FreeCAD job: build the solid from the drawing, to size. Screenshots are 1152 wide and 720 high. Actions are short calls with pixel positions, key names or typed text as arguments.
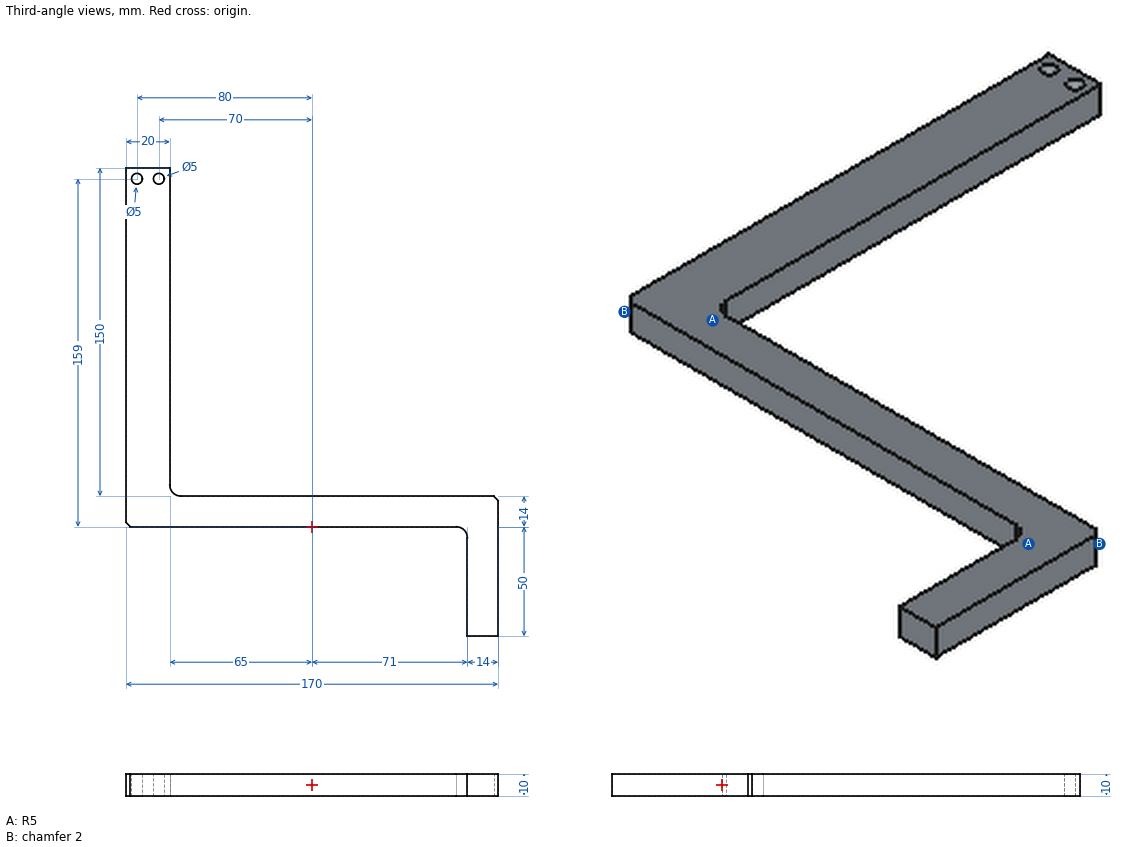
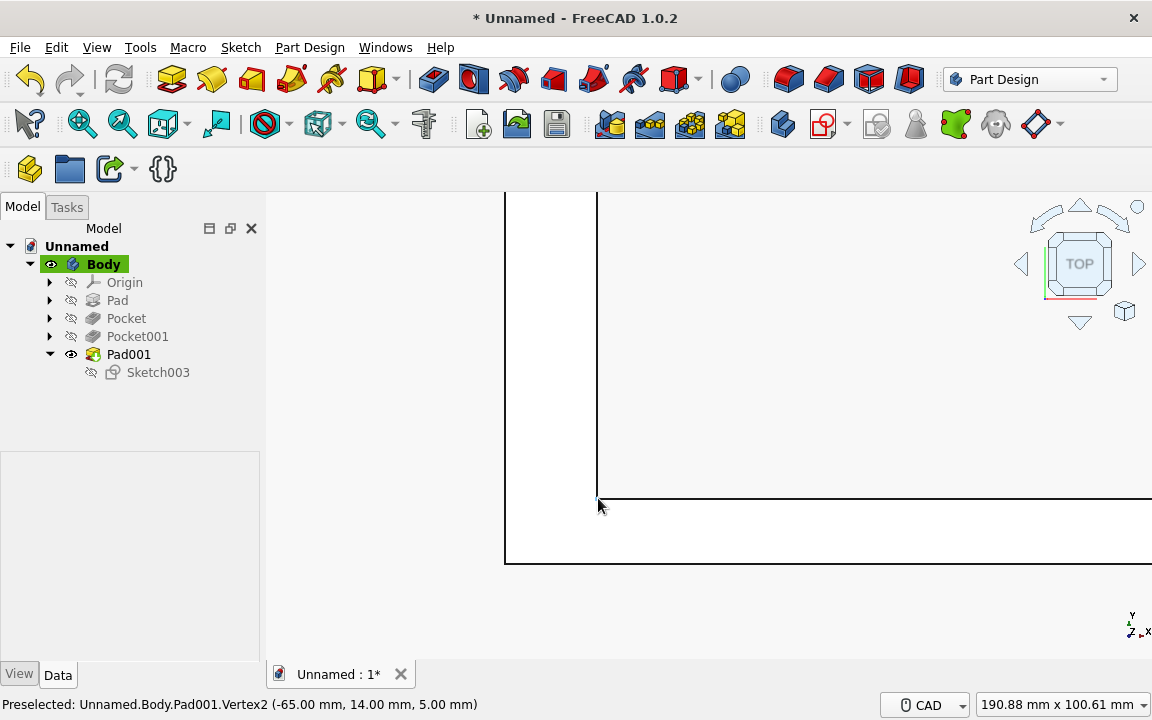
click(84, 124)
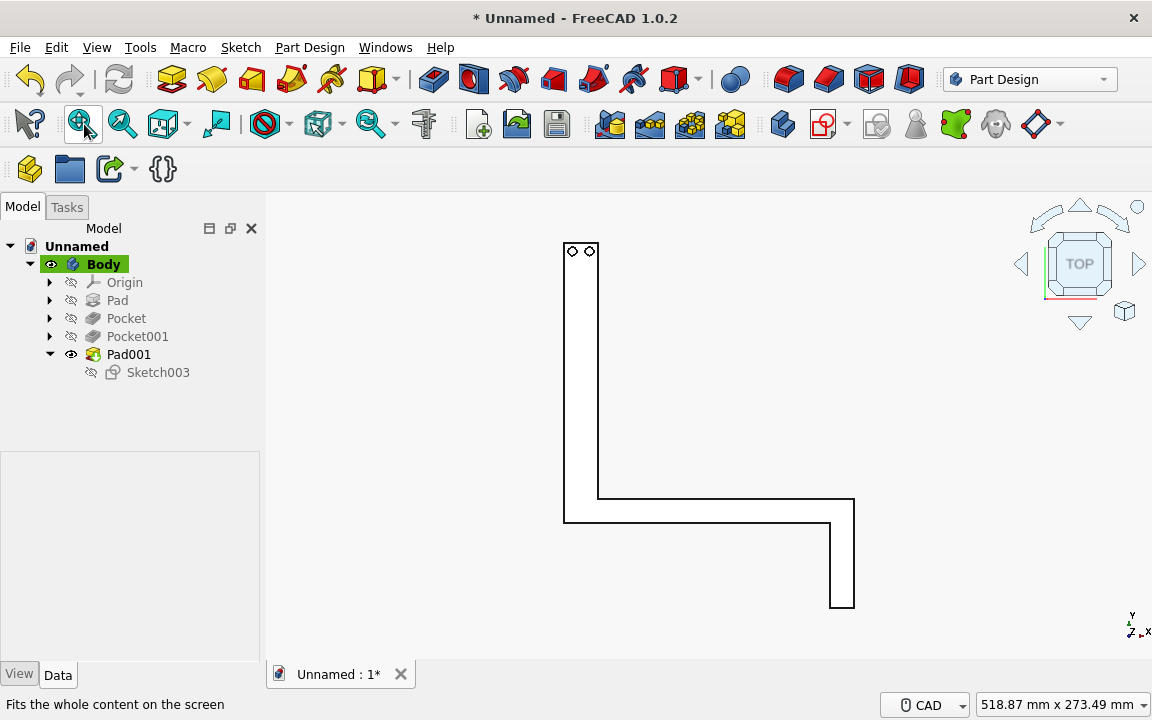
key(1)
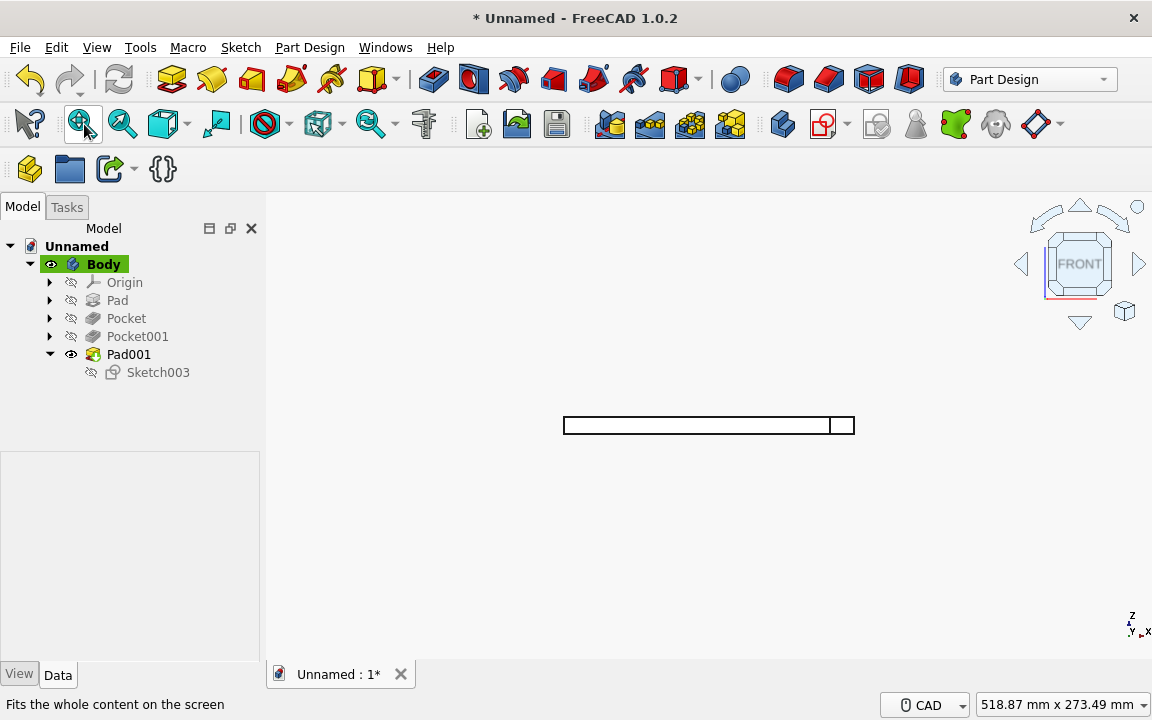
click(84, 124)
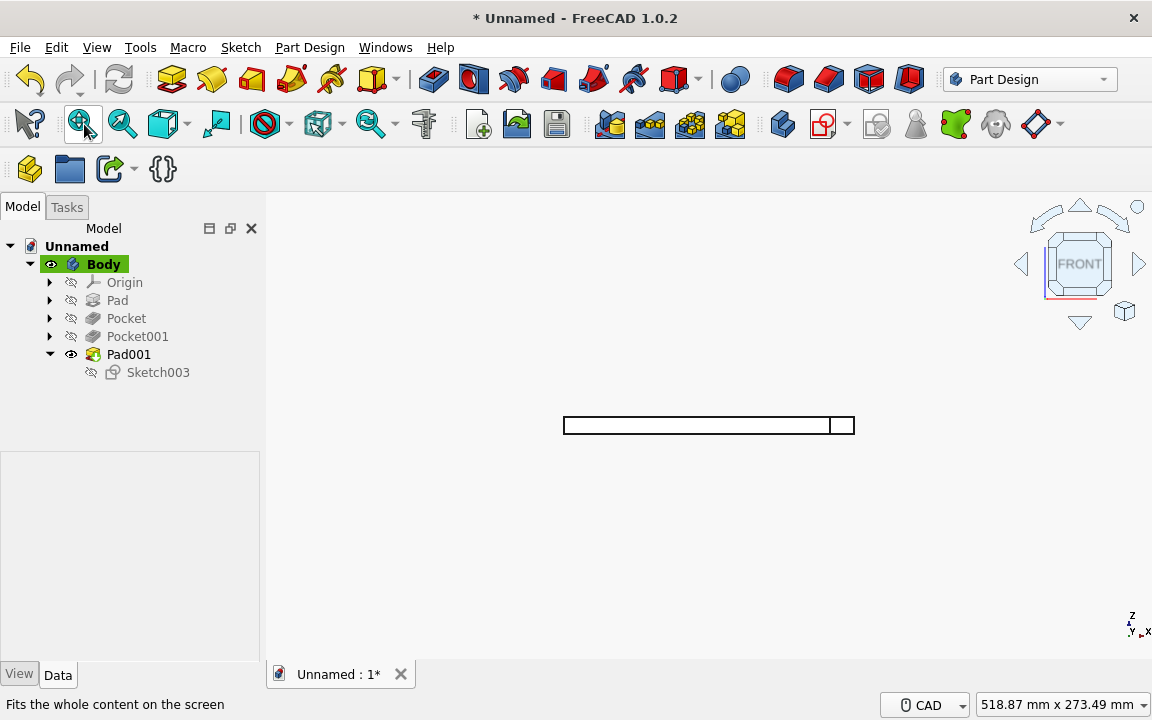
scroll(598, 425, up, 5)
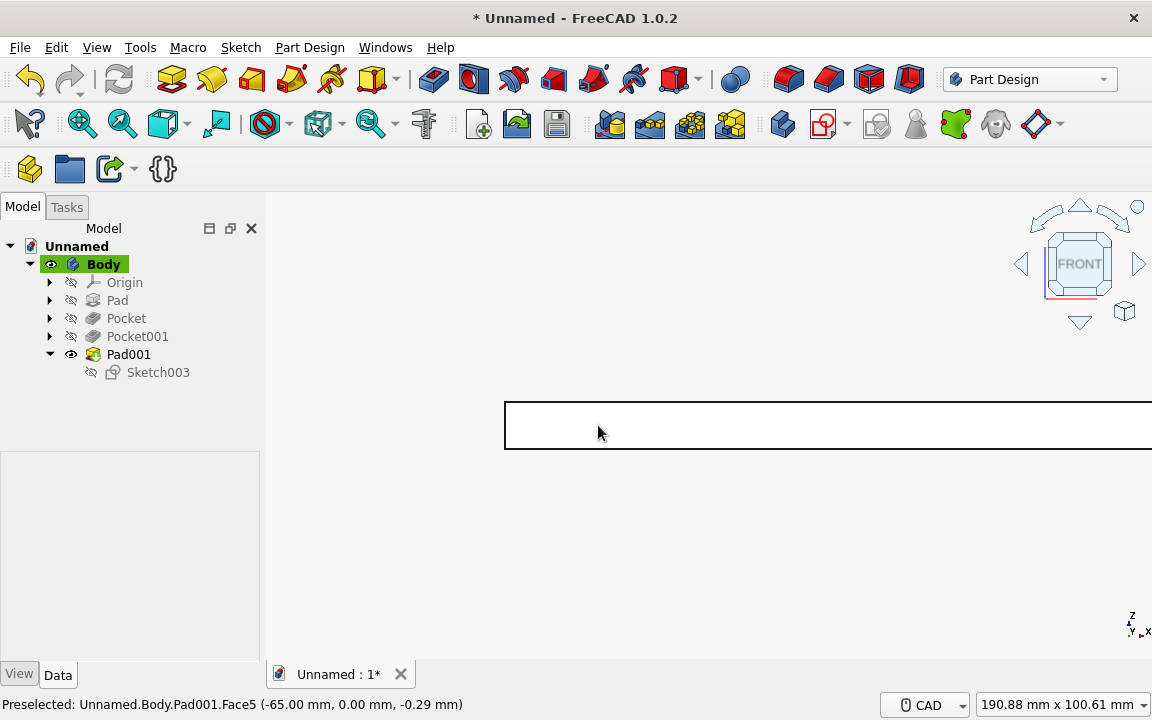
click(84, 124)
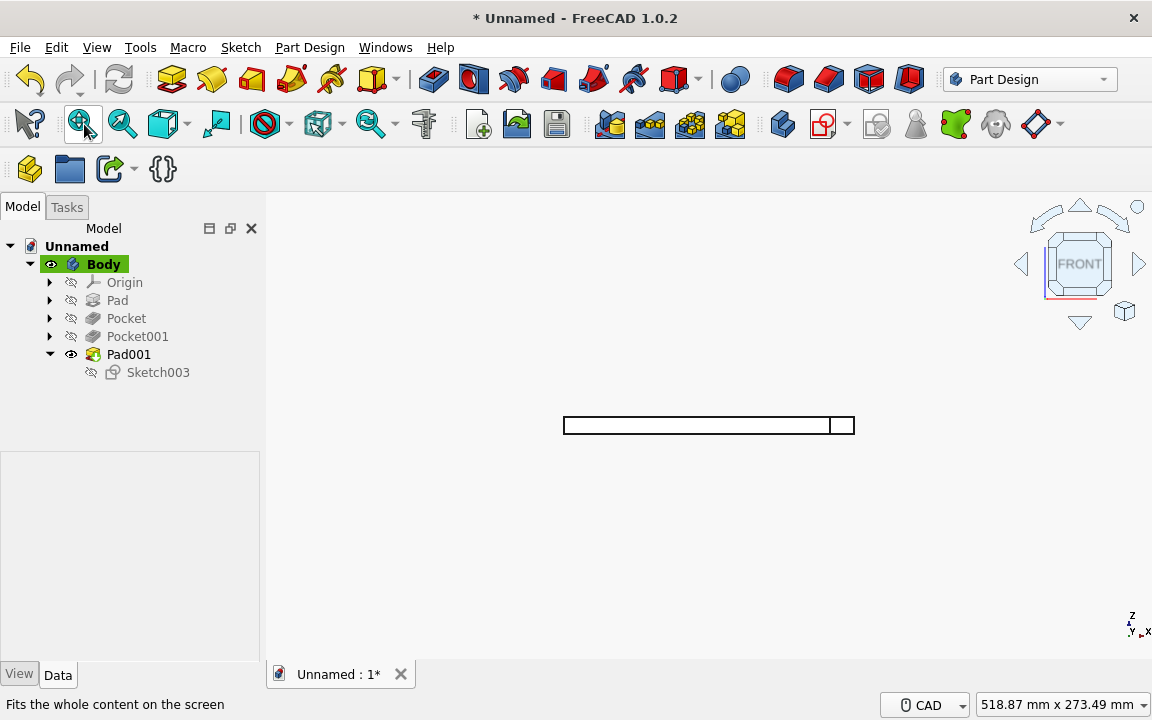
key(3)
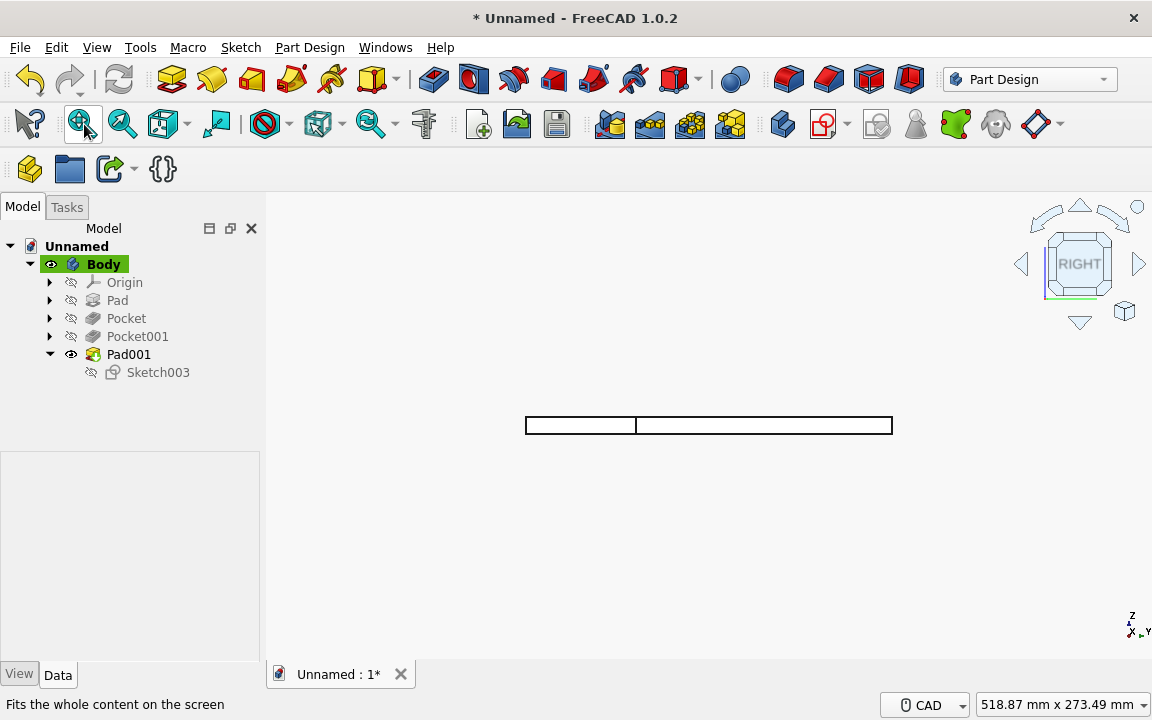
click(84, 124)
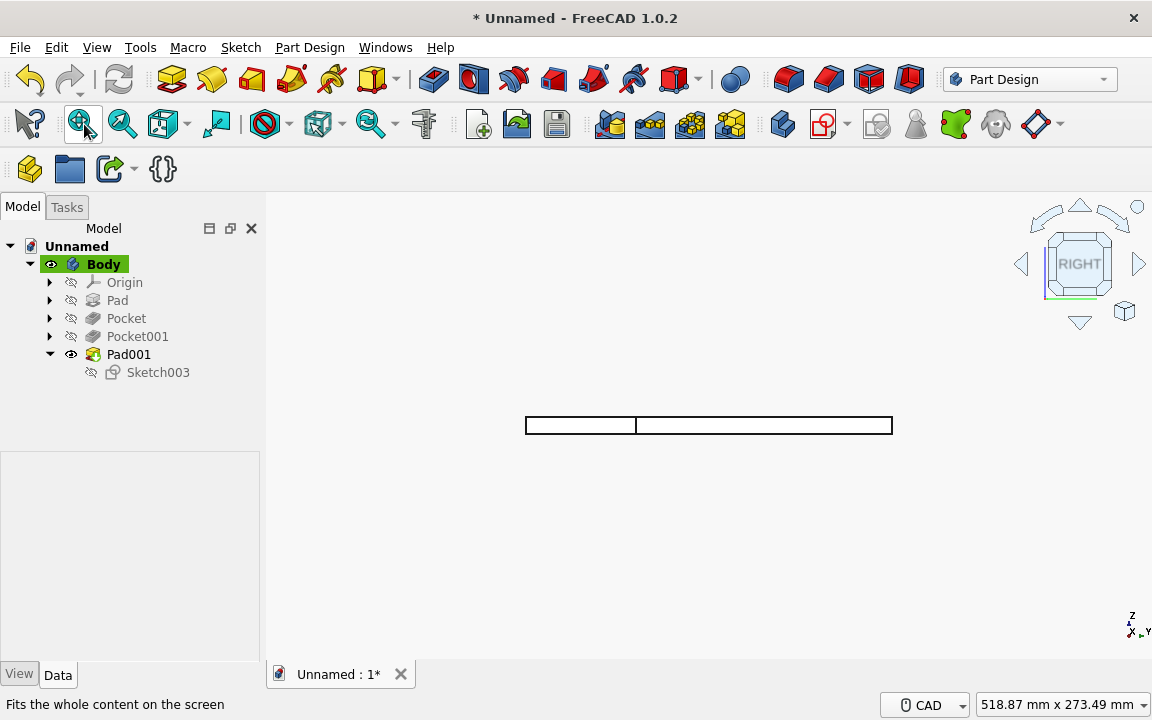
scroll(636, 424, up, 5)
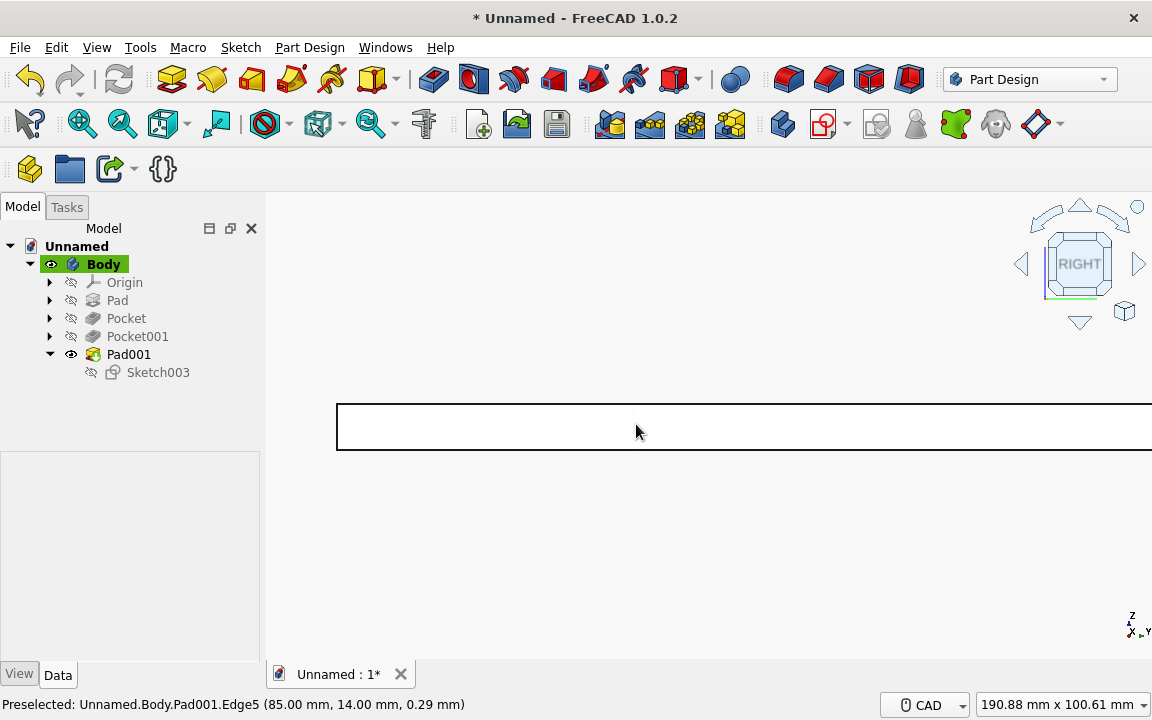
key(v)
key(f)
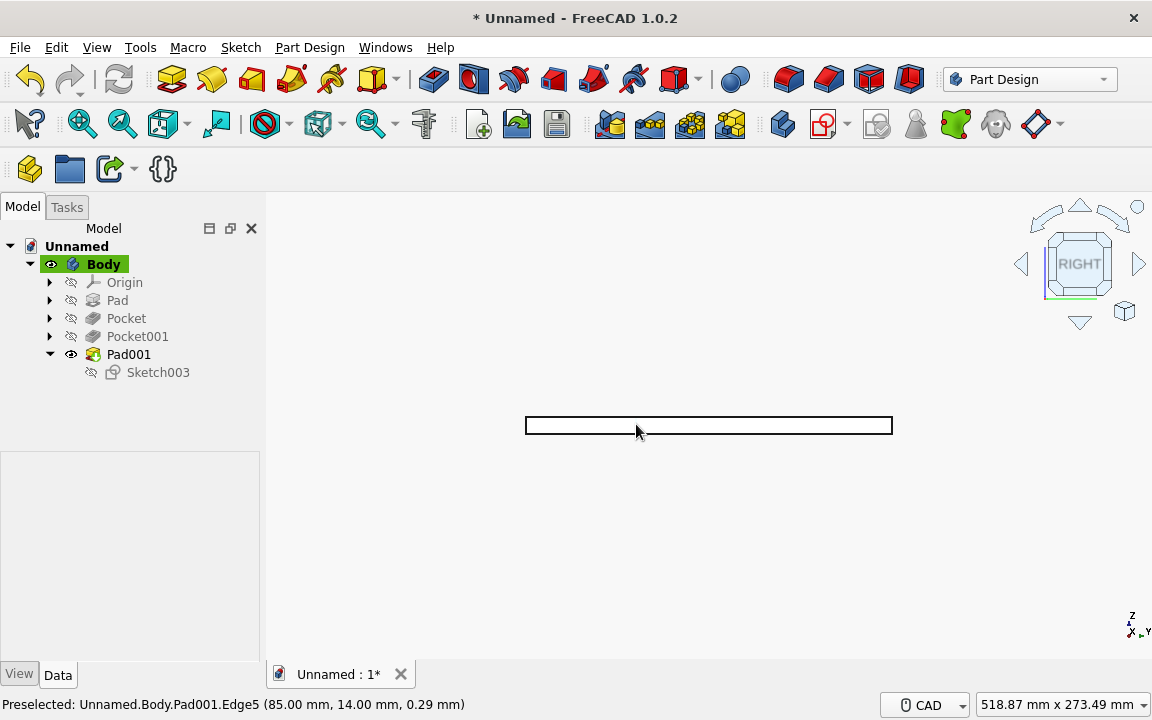
key(5)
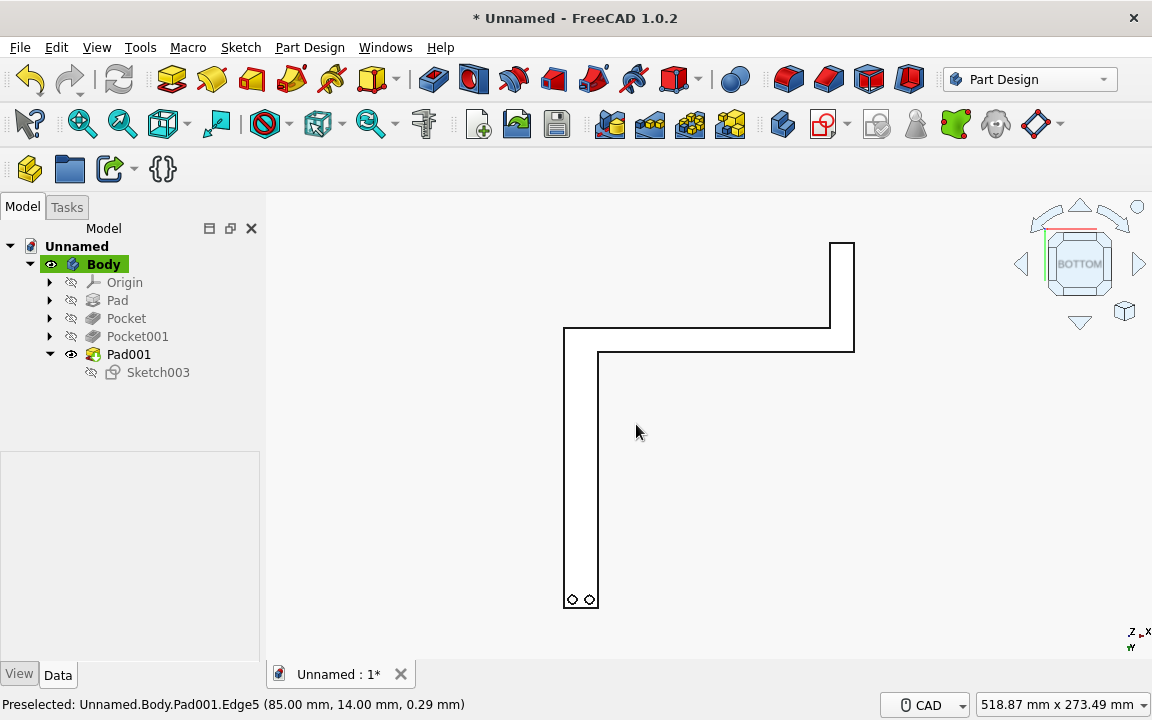
scroll(598, 351, up, 5)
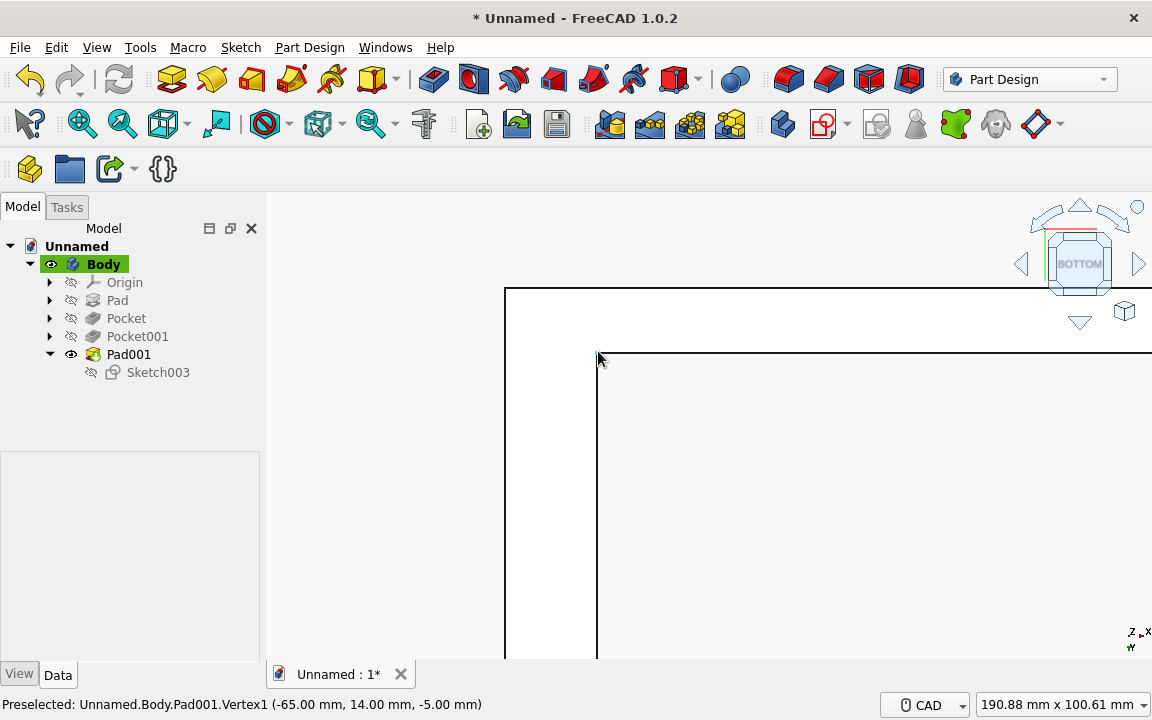
key(v)
key(f)